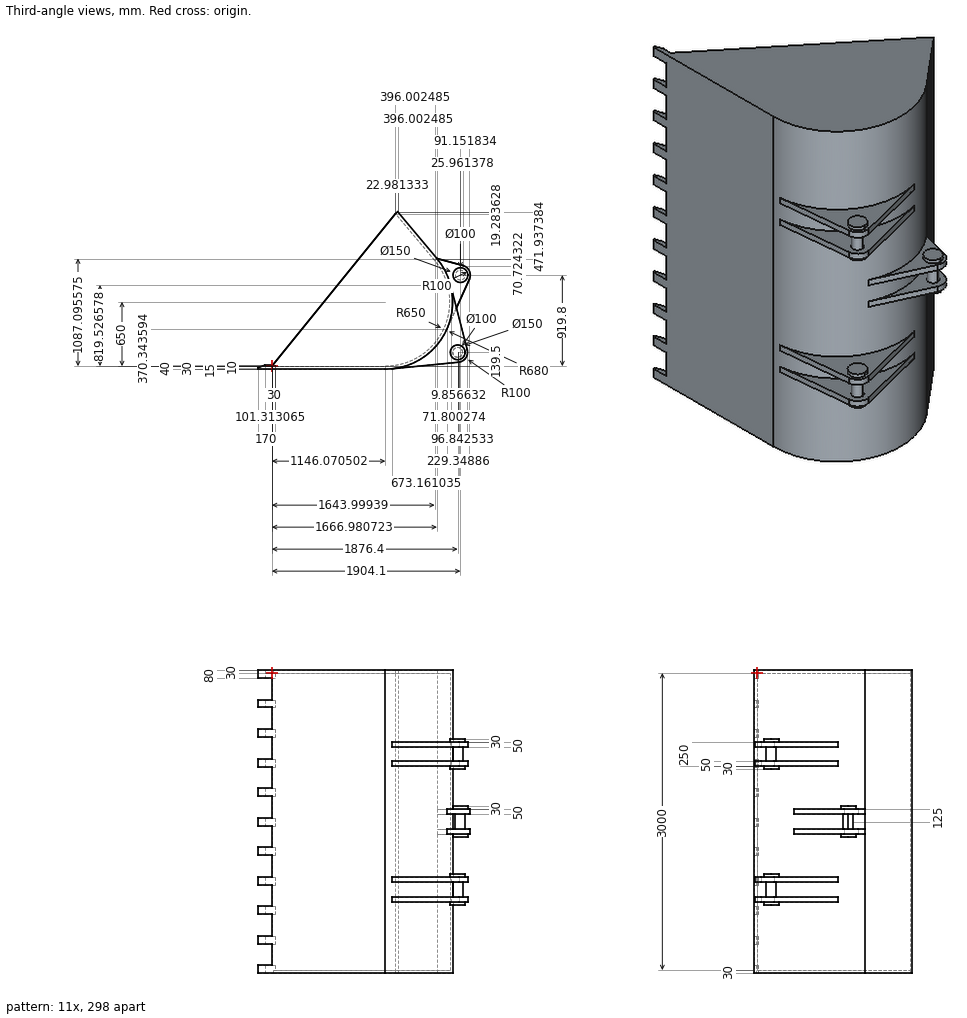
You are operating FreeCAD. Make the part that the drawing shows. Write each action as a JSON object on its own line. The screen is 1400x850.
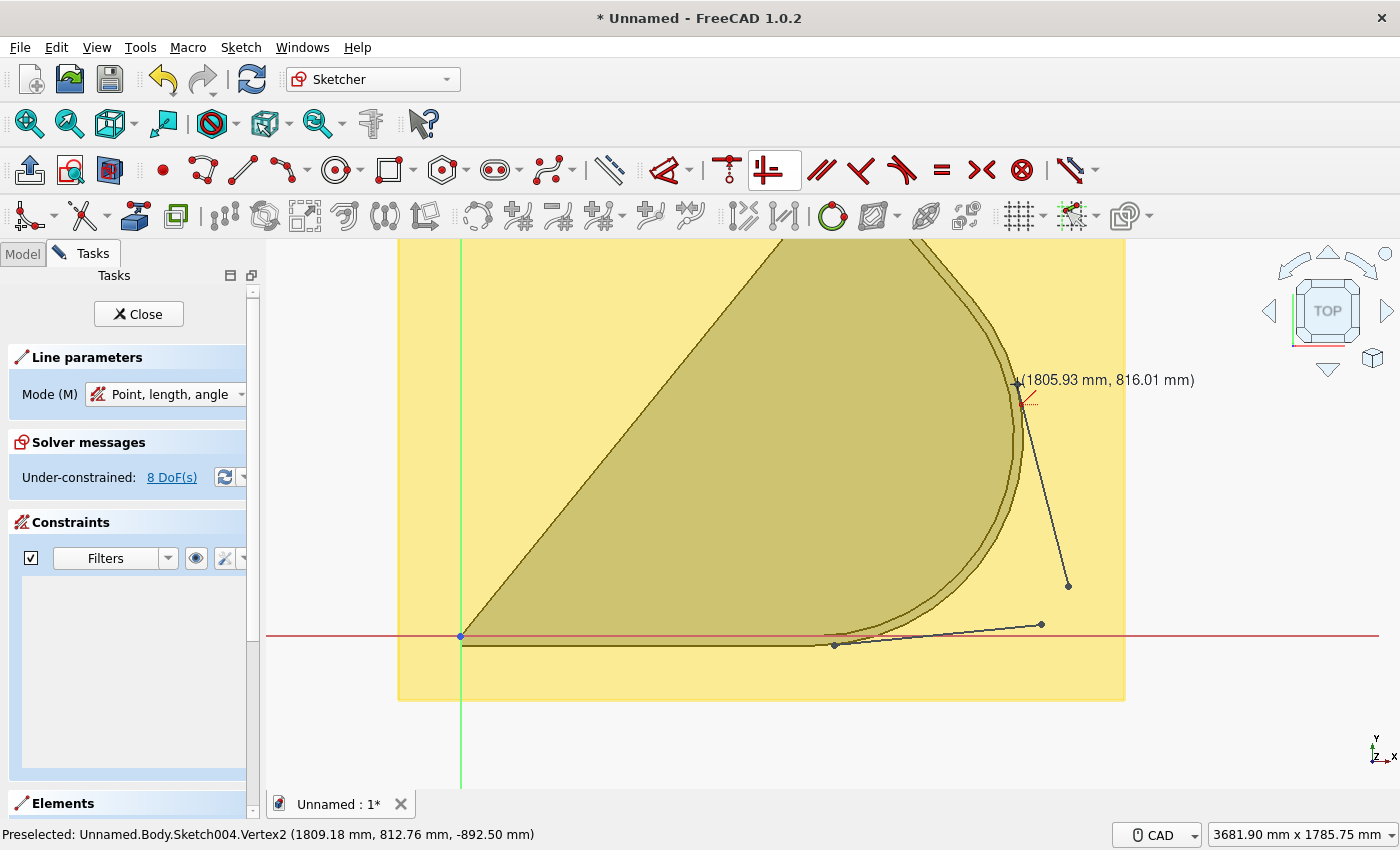
{"action": "left_click", "coordinate": [284, 170]}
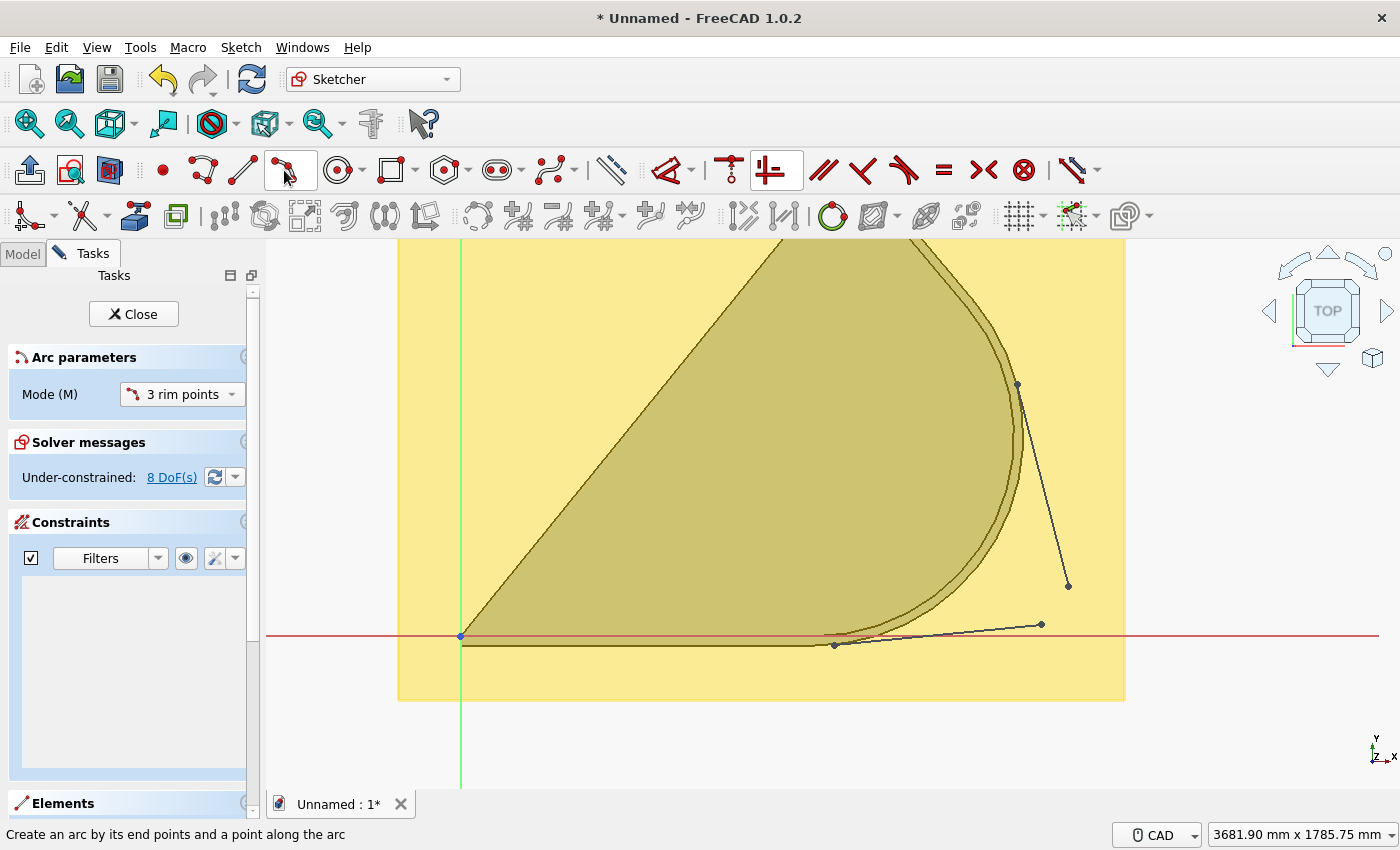
{"action": "scroll", "coordinate": [1042, 624], "scroll_direction": "up", "scroll_amount": 2}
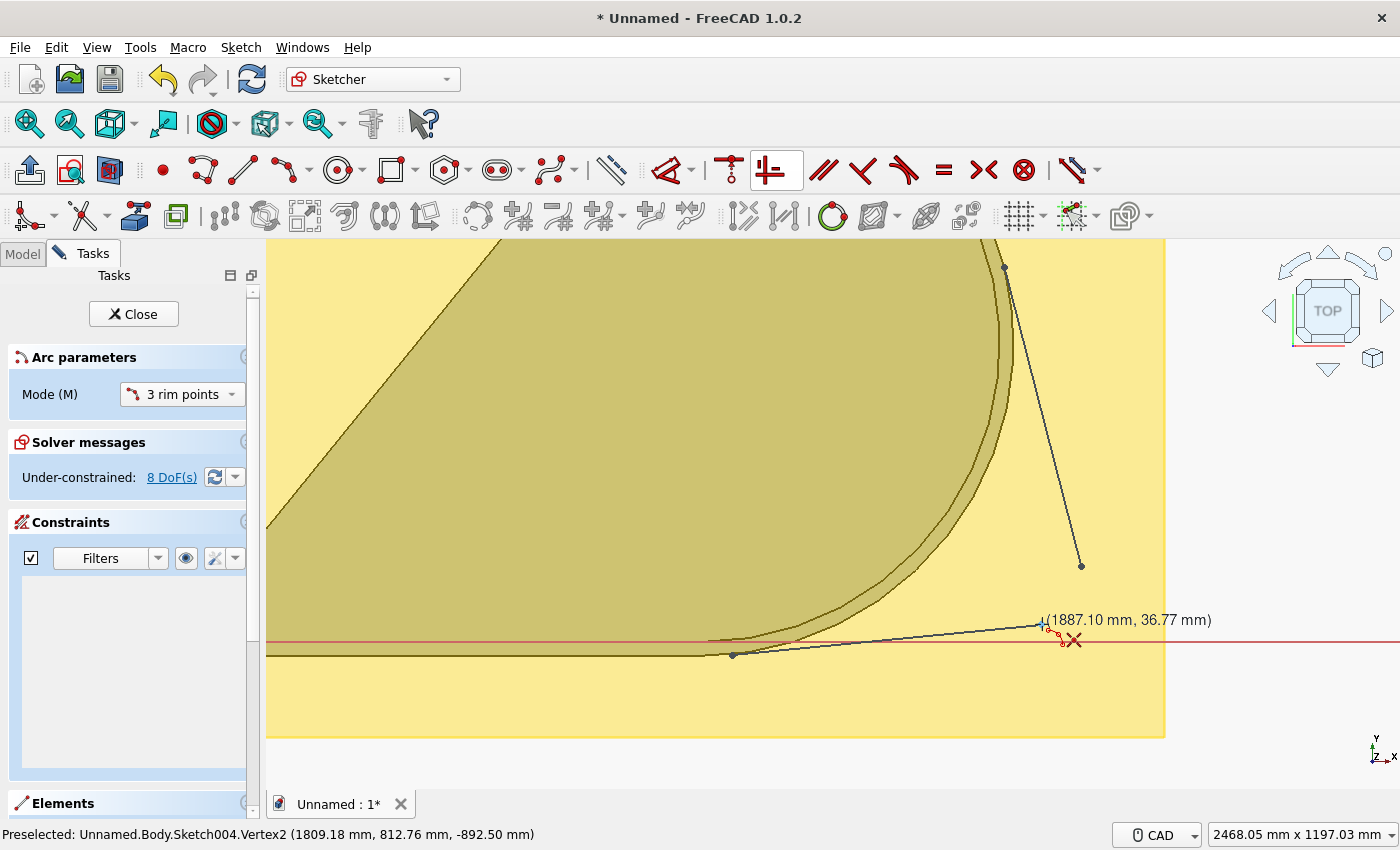
{"action": "left_click", "coordinate": [1042, 625]}
{"action": "left_click", "coordinate": [1082, 567]}
{"action": "left_click", "coordinate": [1074, 604]}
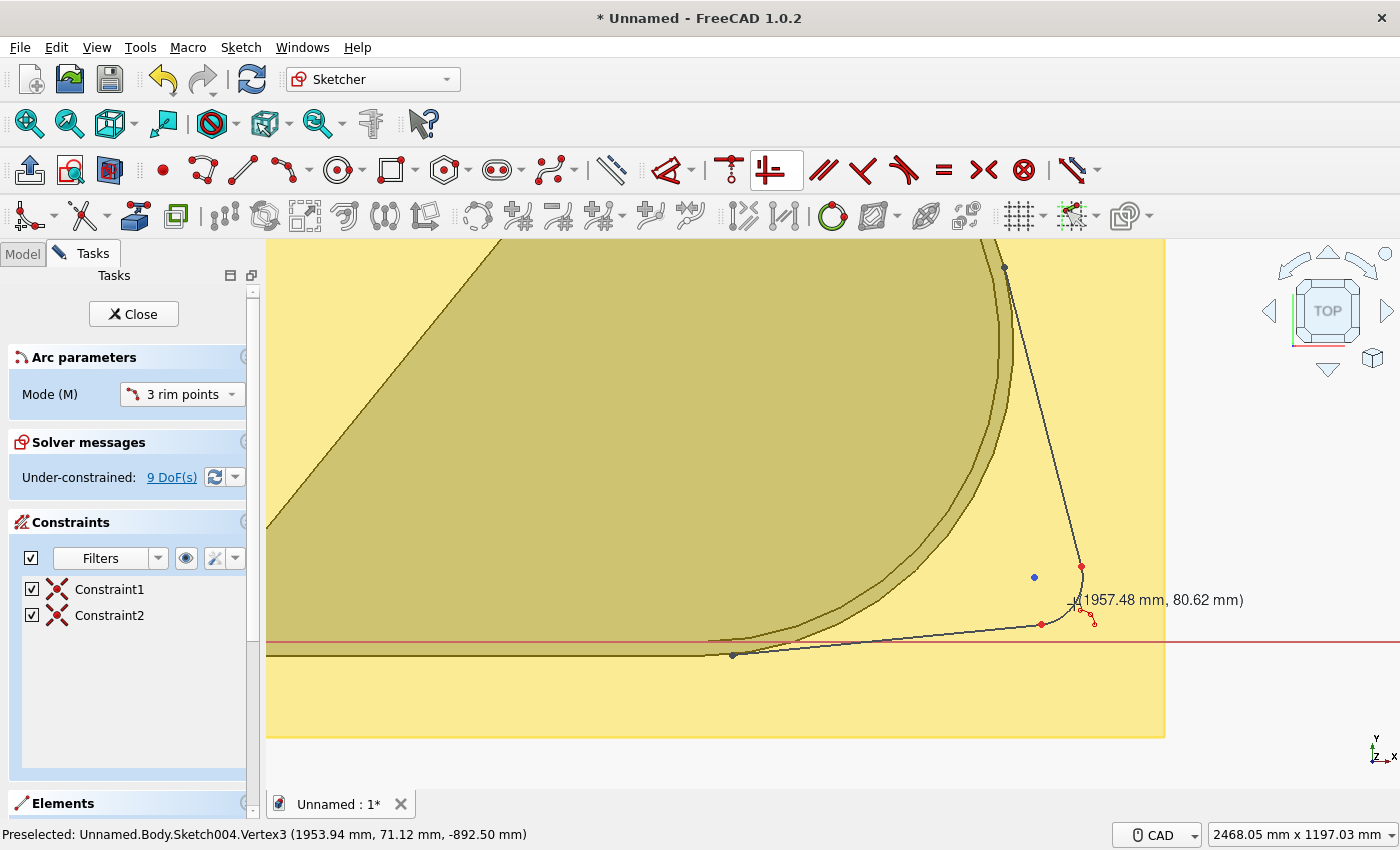
{"action": "scroll", "coordinate": [1042, 624], "scroll_direction": "down", "scroll_amount": 2}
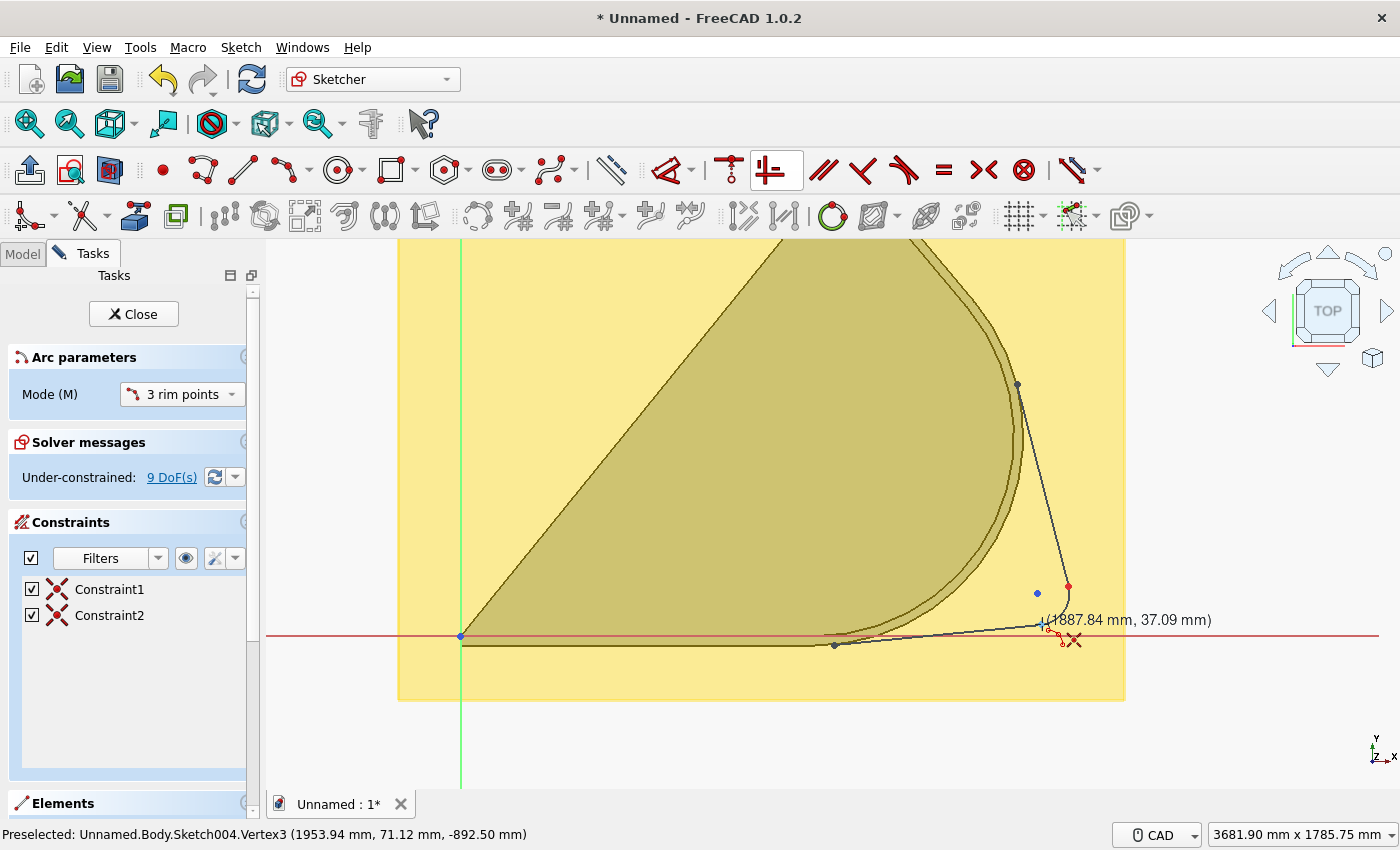
{"action": "left_click", "coordinate": [1017, 385]}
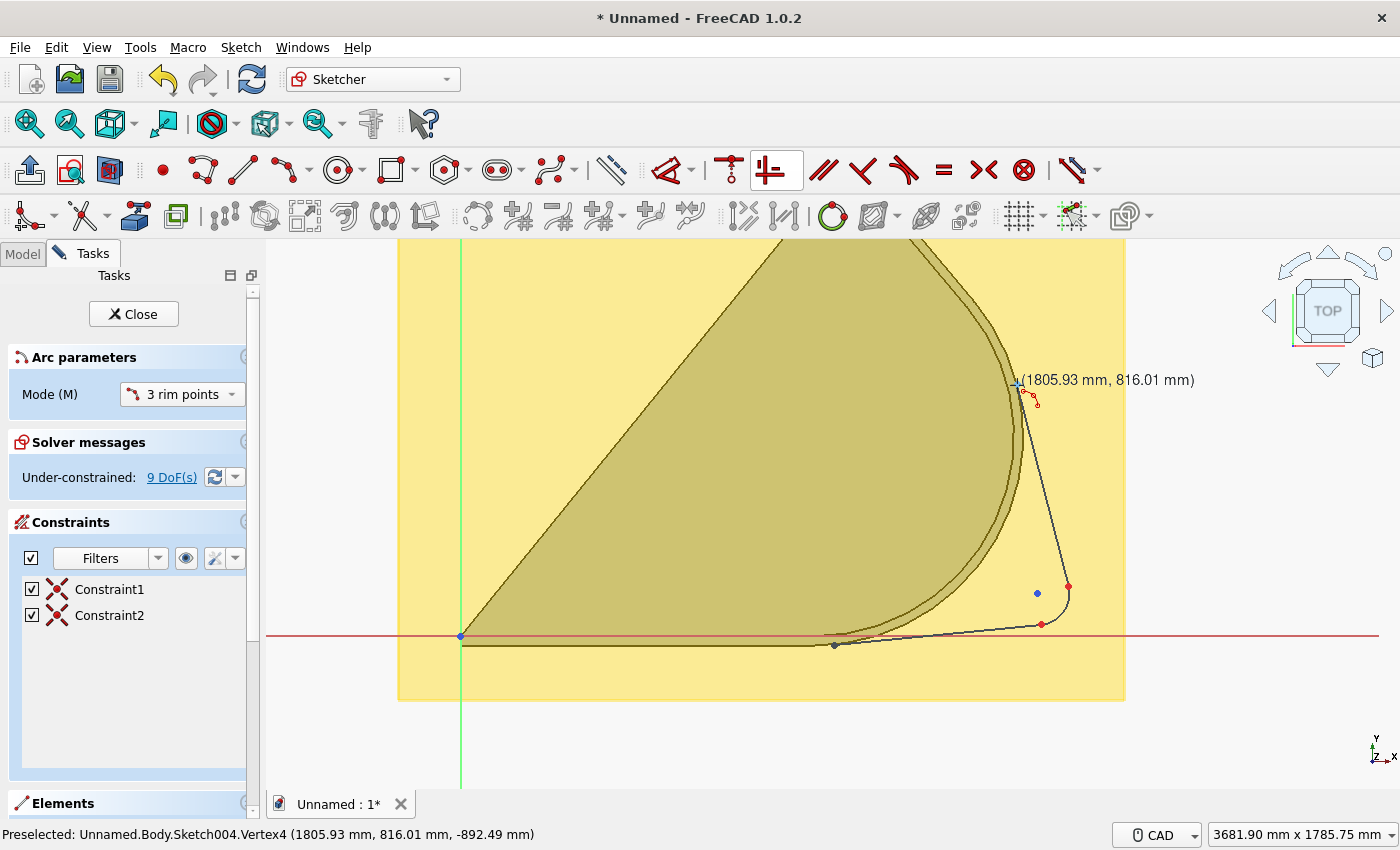
{"action": "scroll", "coordinate": [834, 645], "scroll_direction": "up", "scroll_amount": 4}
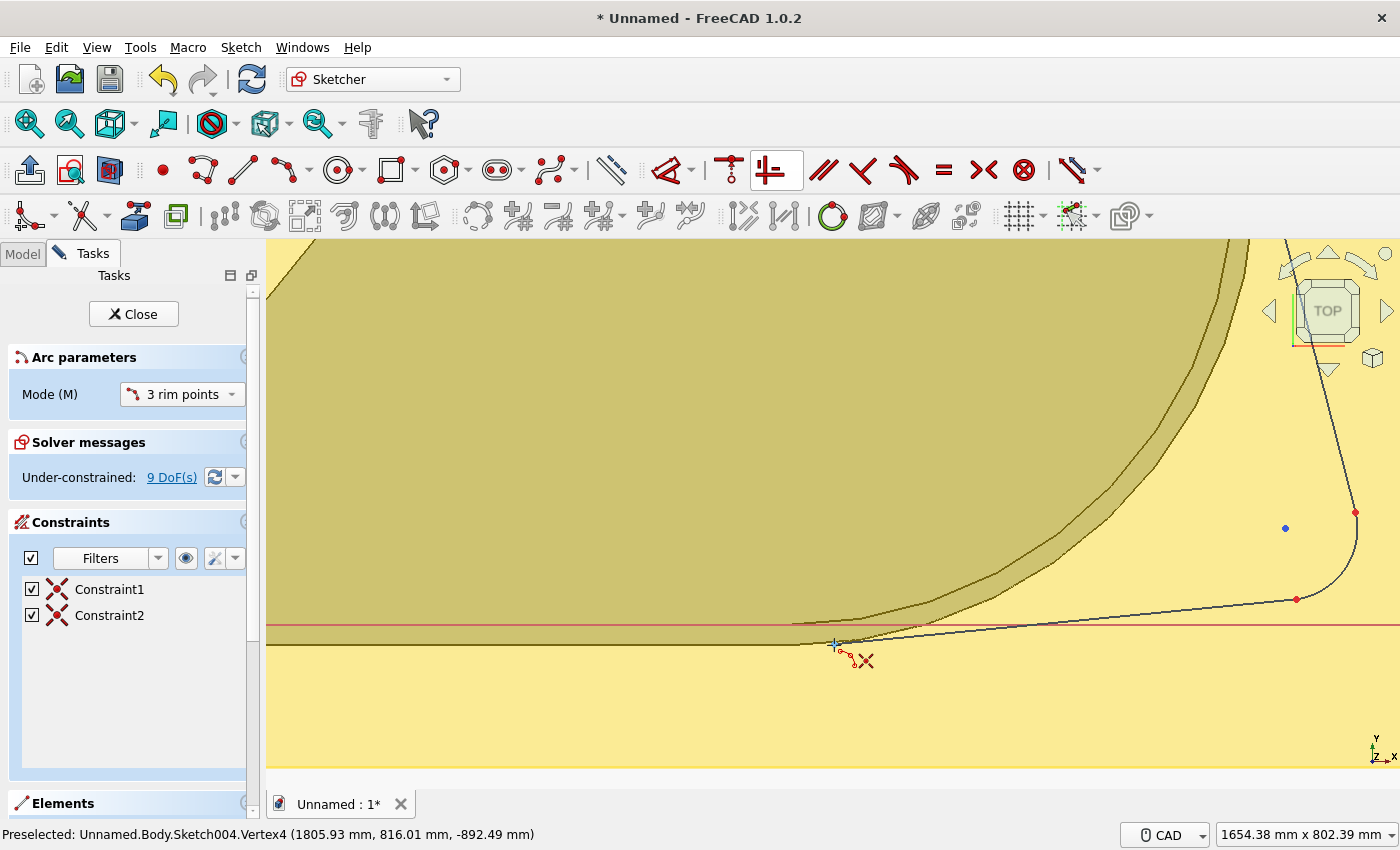
{"action": "left_click", "coordinate": [834, 644]}
{"action": "left_click", "coordinate": [1170, 446]}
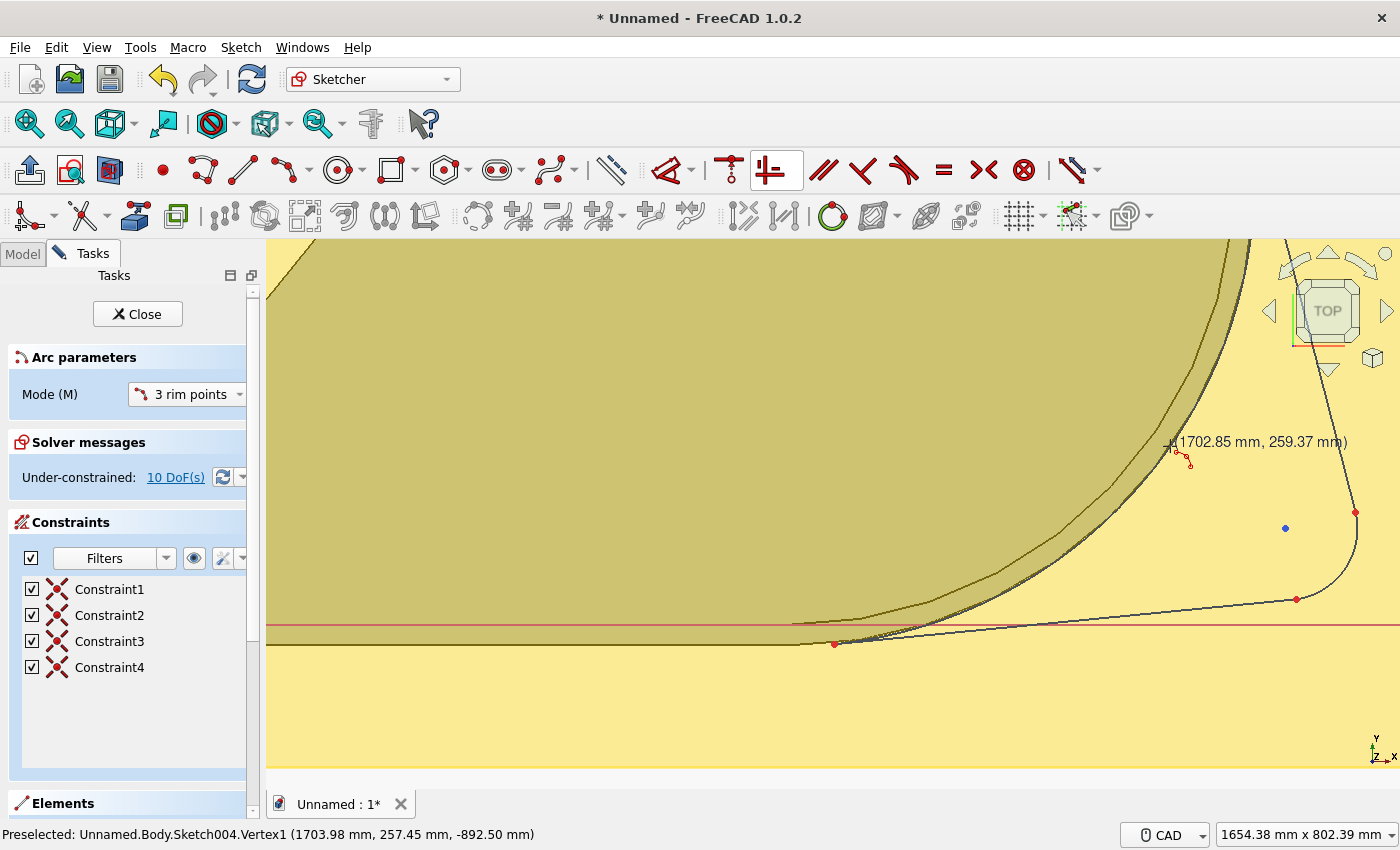
{"action": "left_click", "coordinate": [338, 170]}